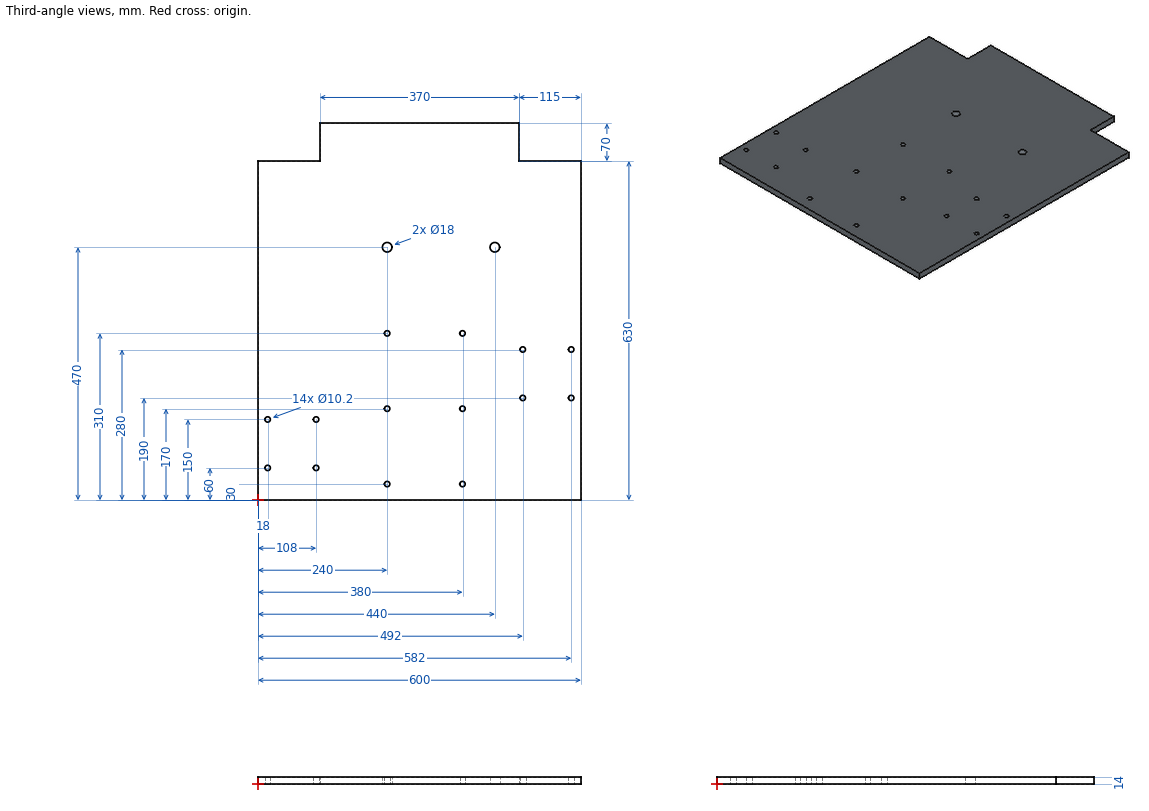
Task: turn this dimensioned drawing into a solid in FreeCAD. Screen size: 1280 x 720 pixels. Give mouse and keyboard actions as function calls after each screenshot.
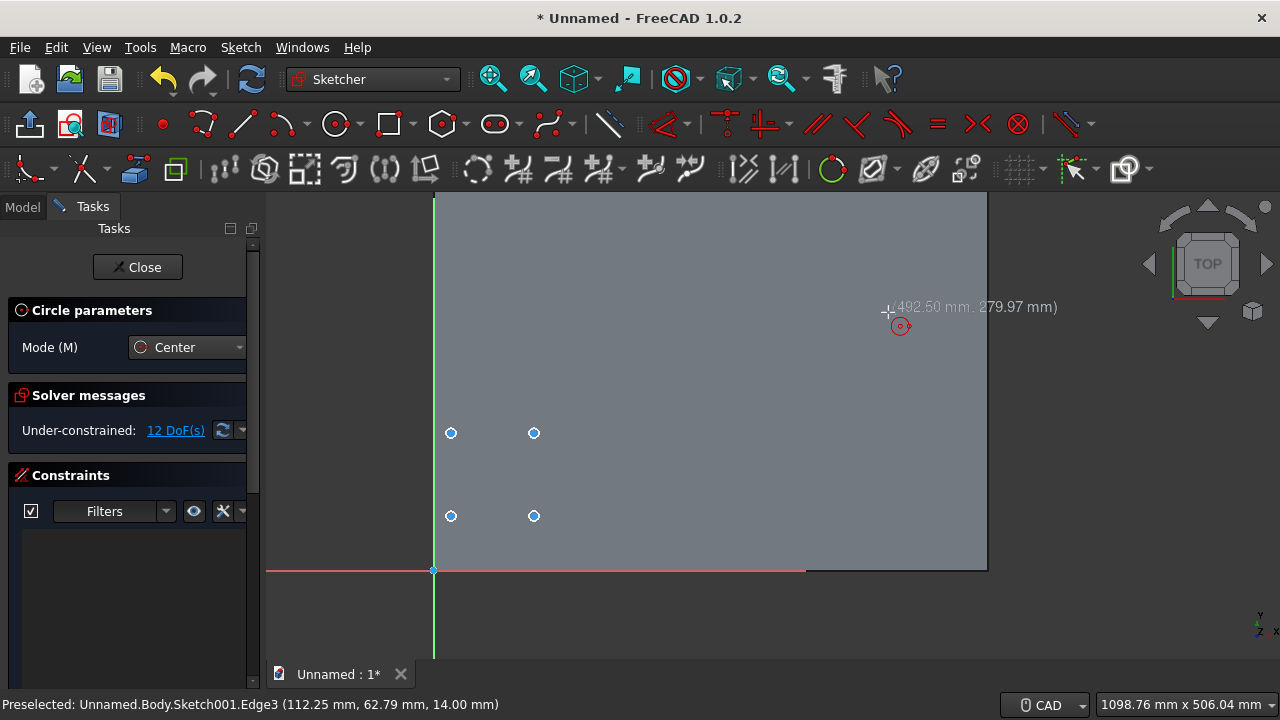
click(888, 312)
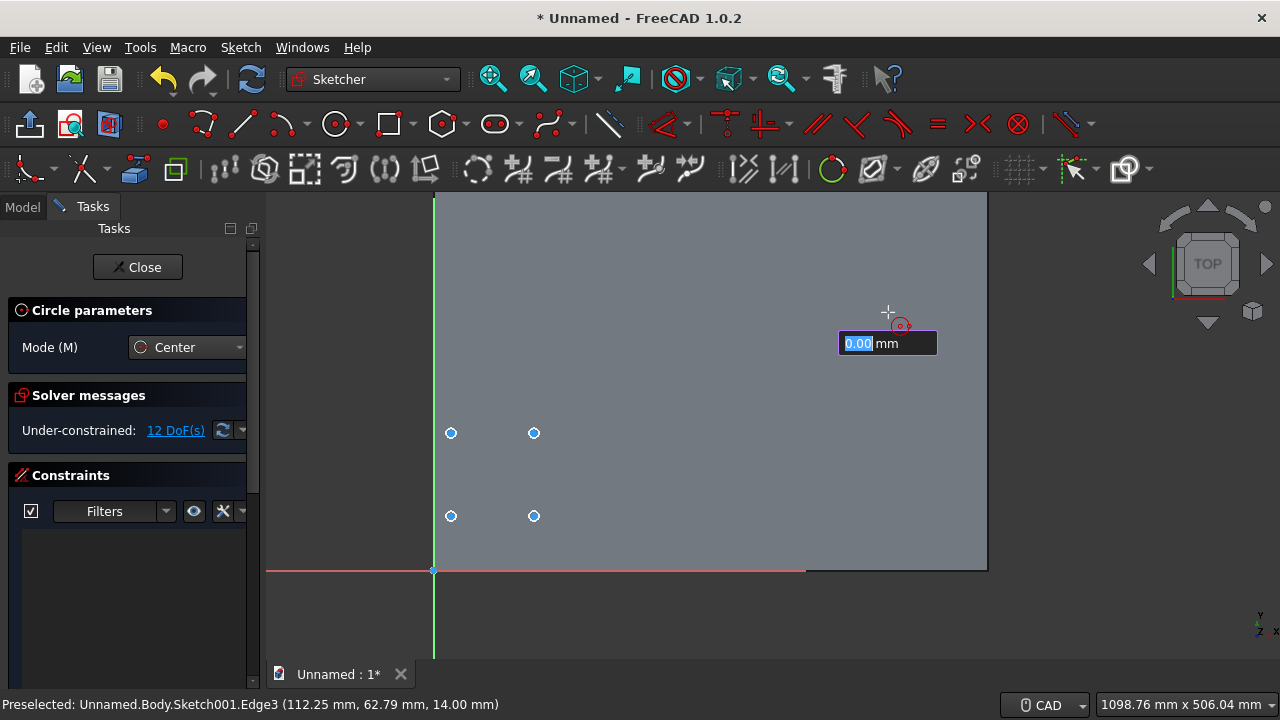
scroll(891, 309, up, 7)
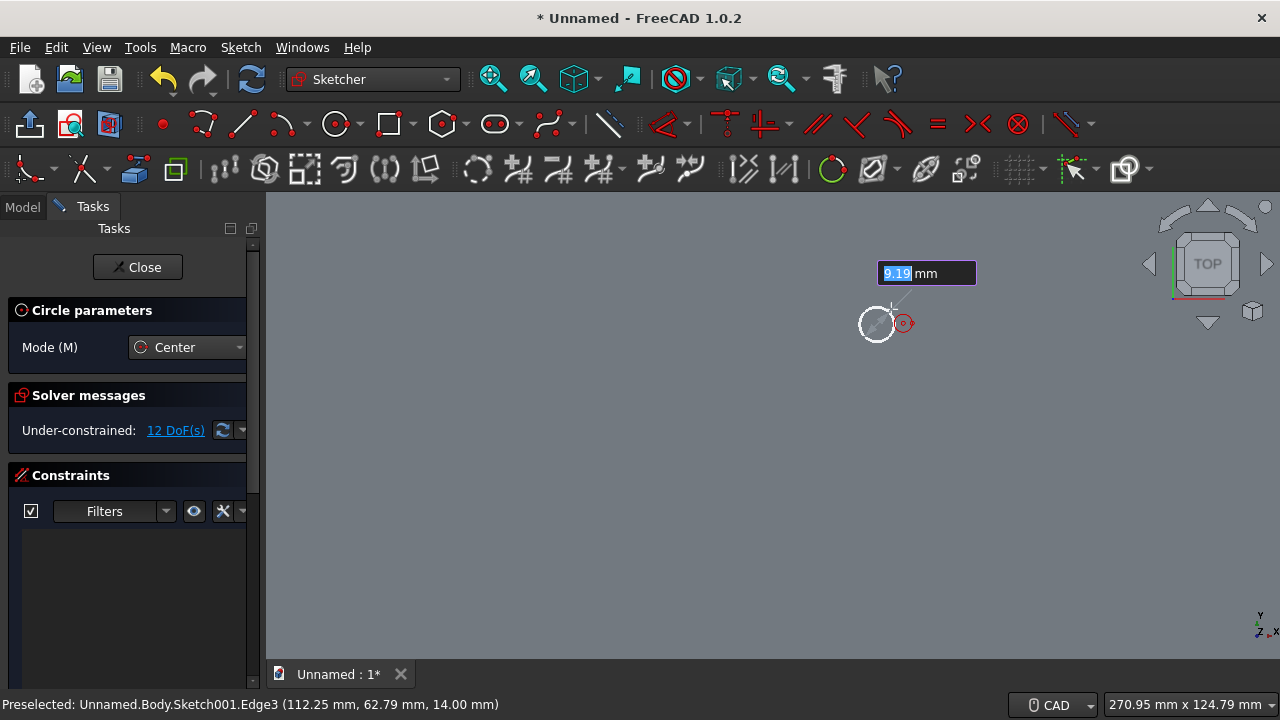
click(891, 308)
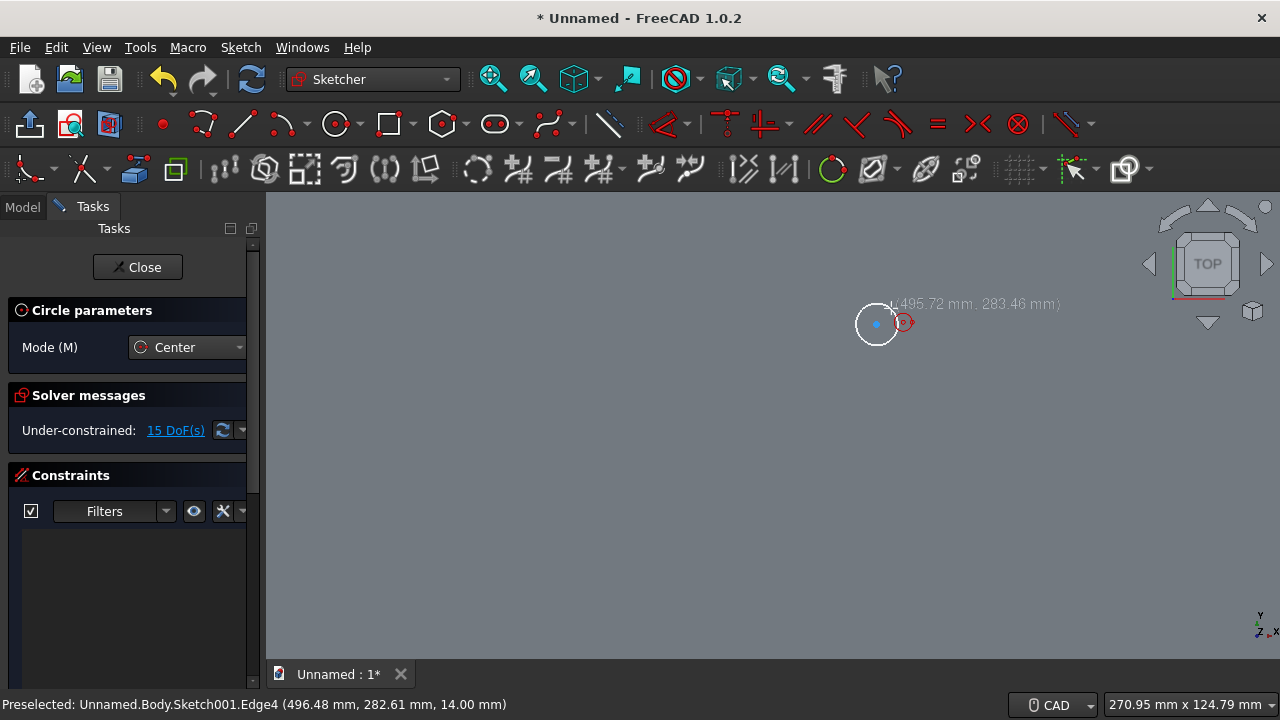
scroll(891, 309, down, 7)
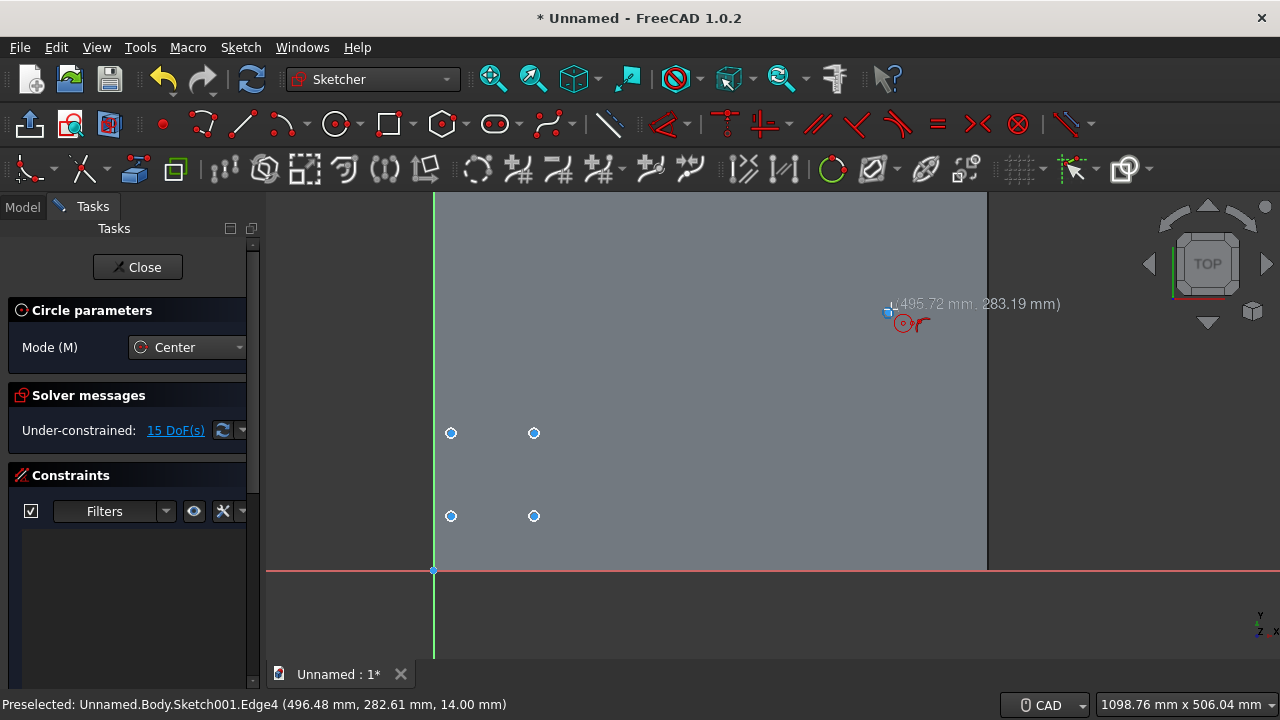
scroll(971, 312, up, 8)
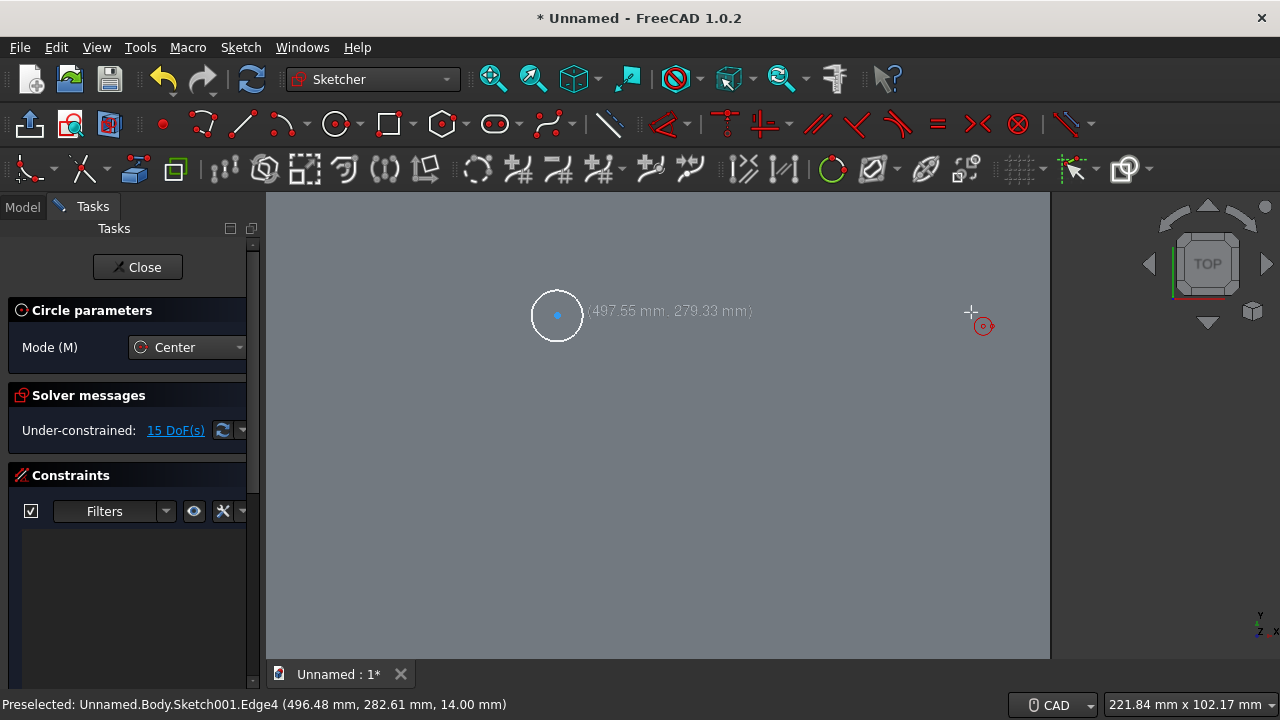
scroll(971, 312, down, 8)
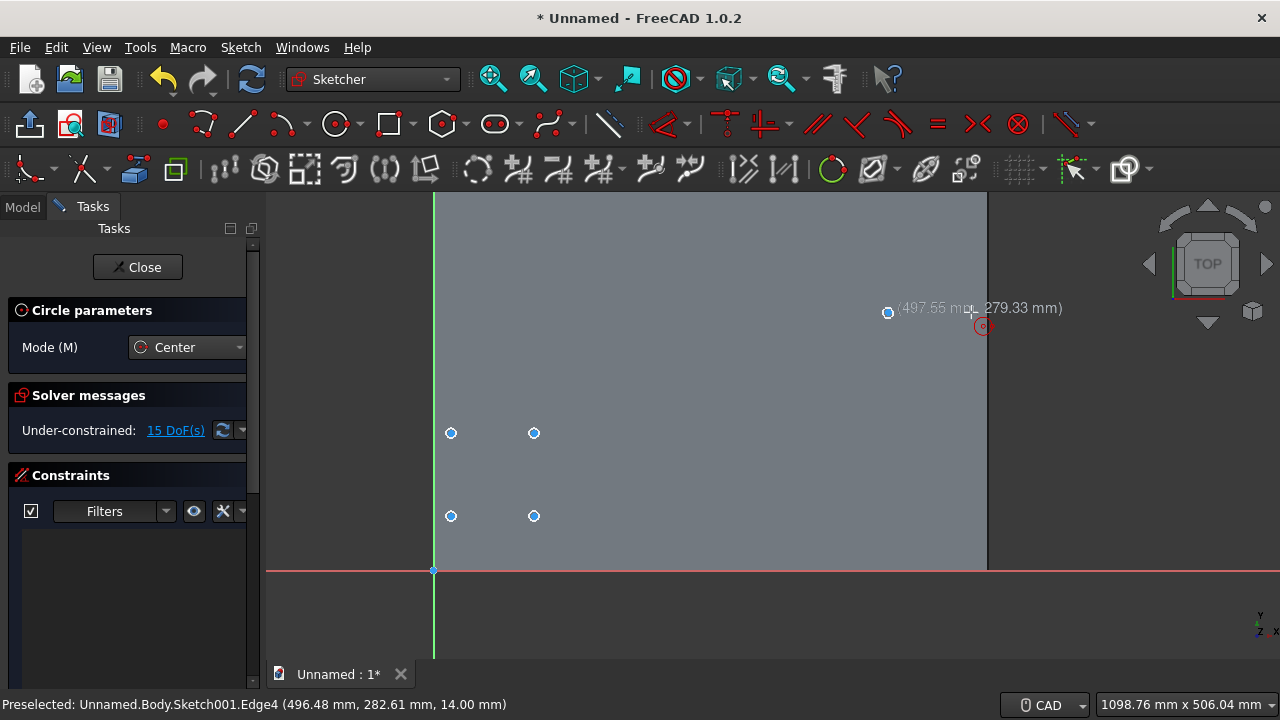
click(971, 312)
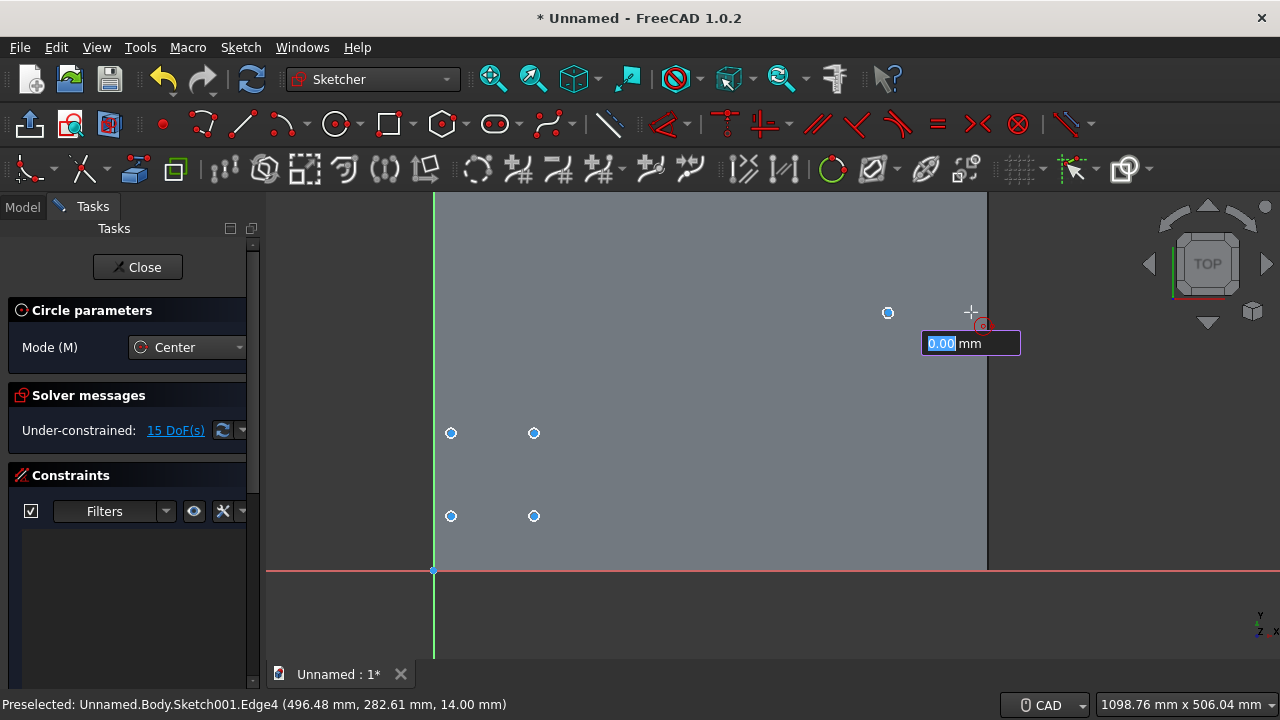
scroll(974, 309, up, 7)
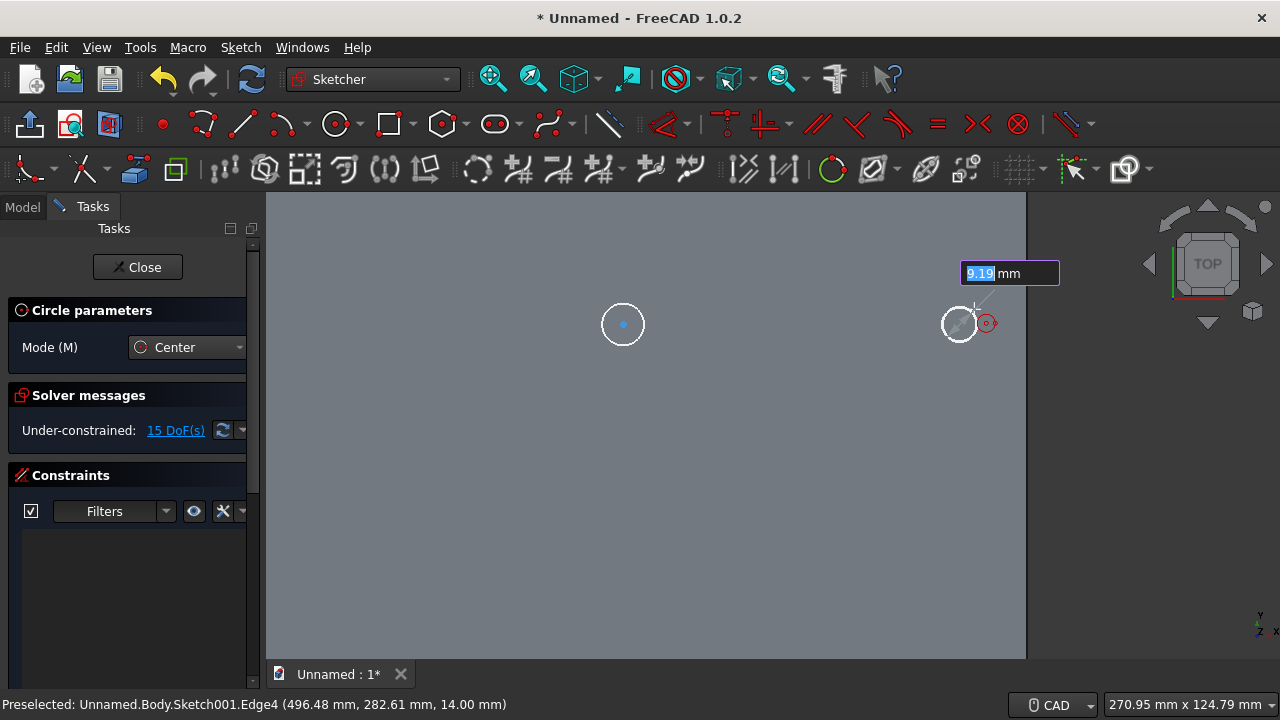
click(974, 308)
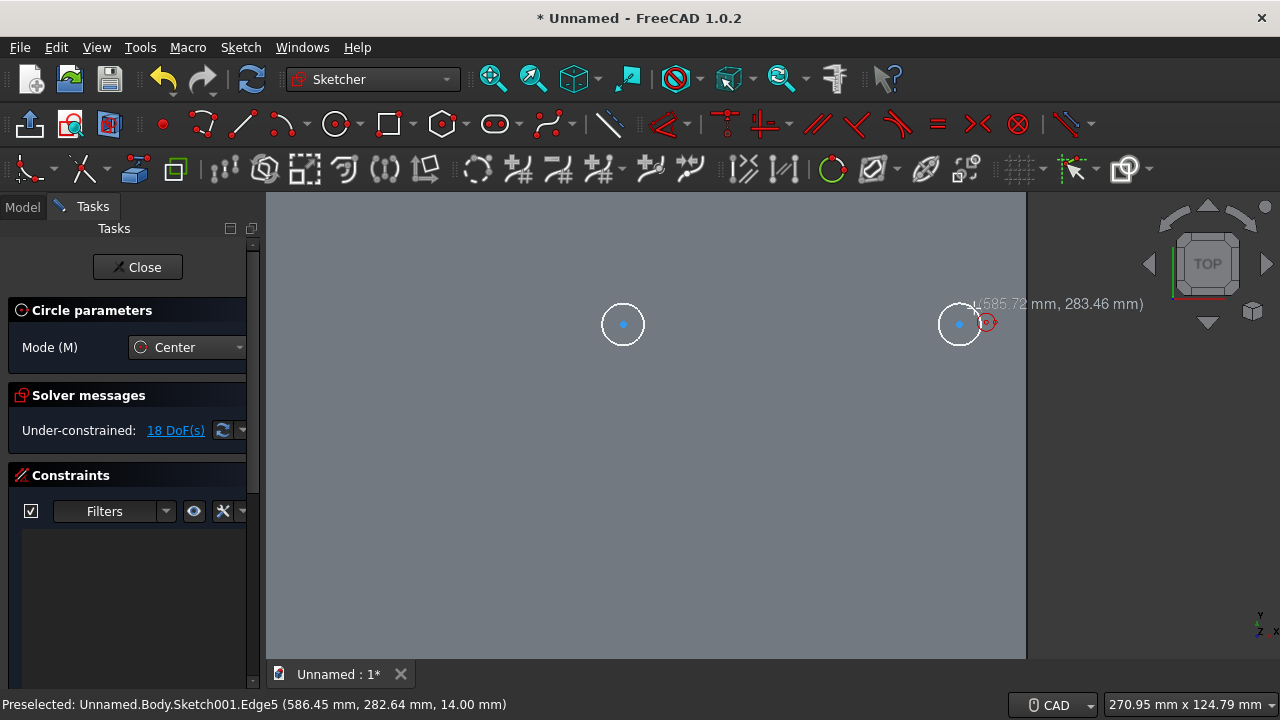
scroll(974, 309, down, 7)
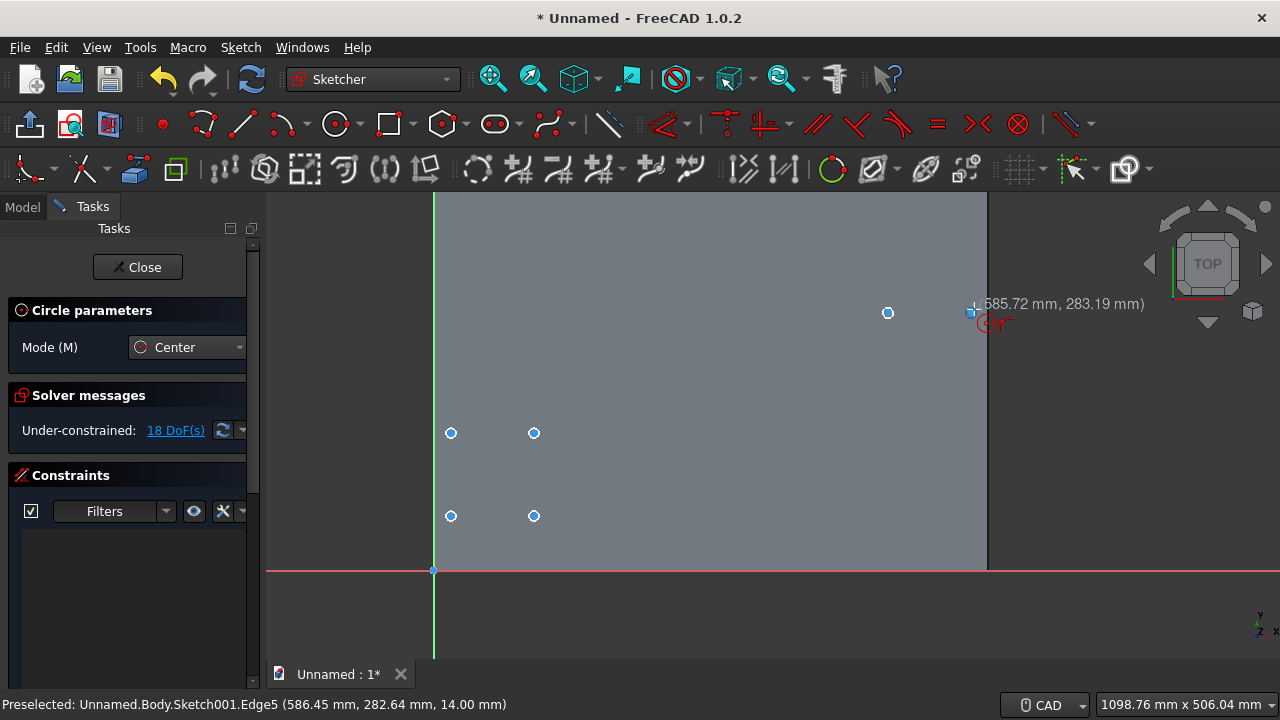
scroll(888, 395, up, 8)